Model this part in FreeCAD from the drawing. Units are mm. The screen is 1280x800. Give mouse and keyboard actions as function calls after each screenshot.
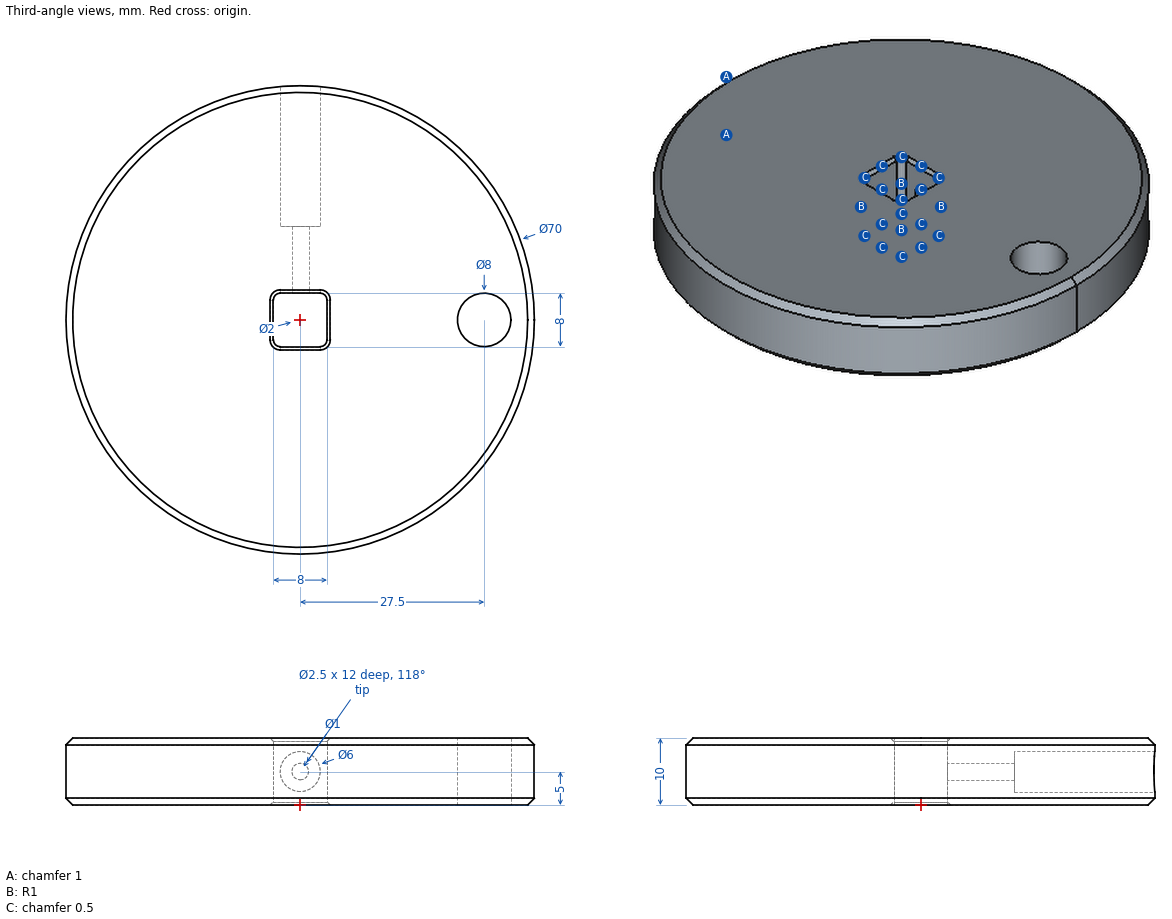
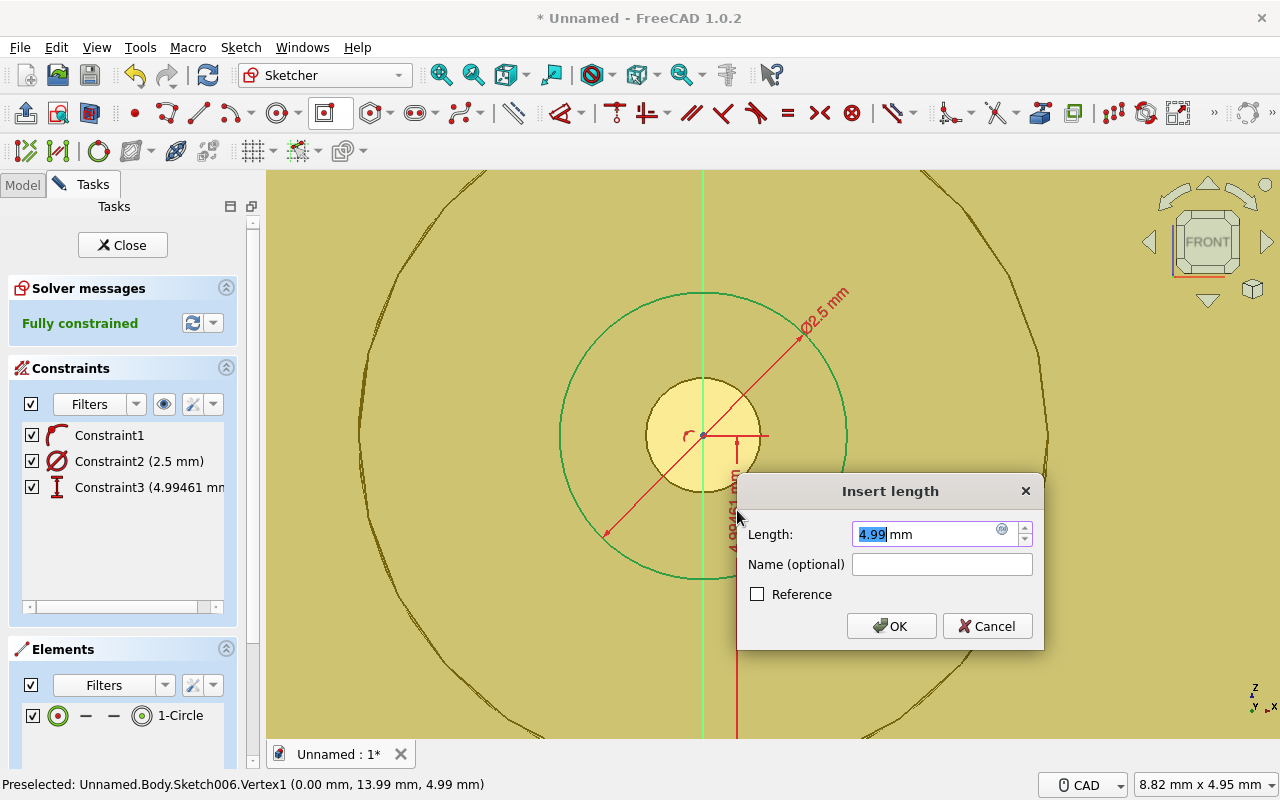
text(5)
key(Return)
key(Escape)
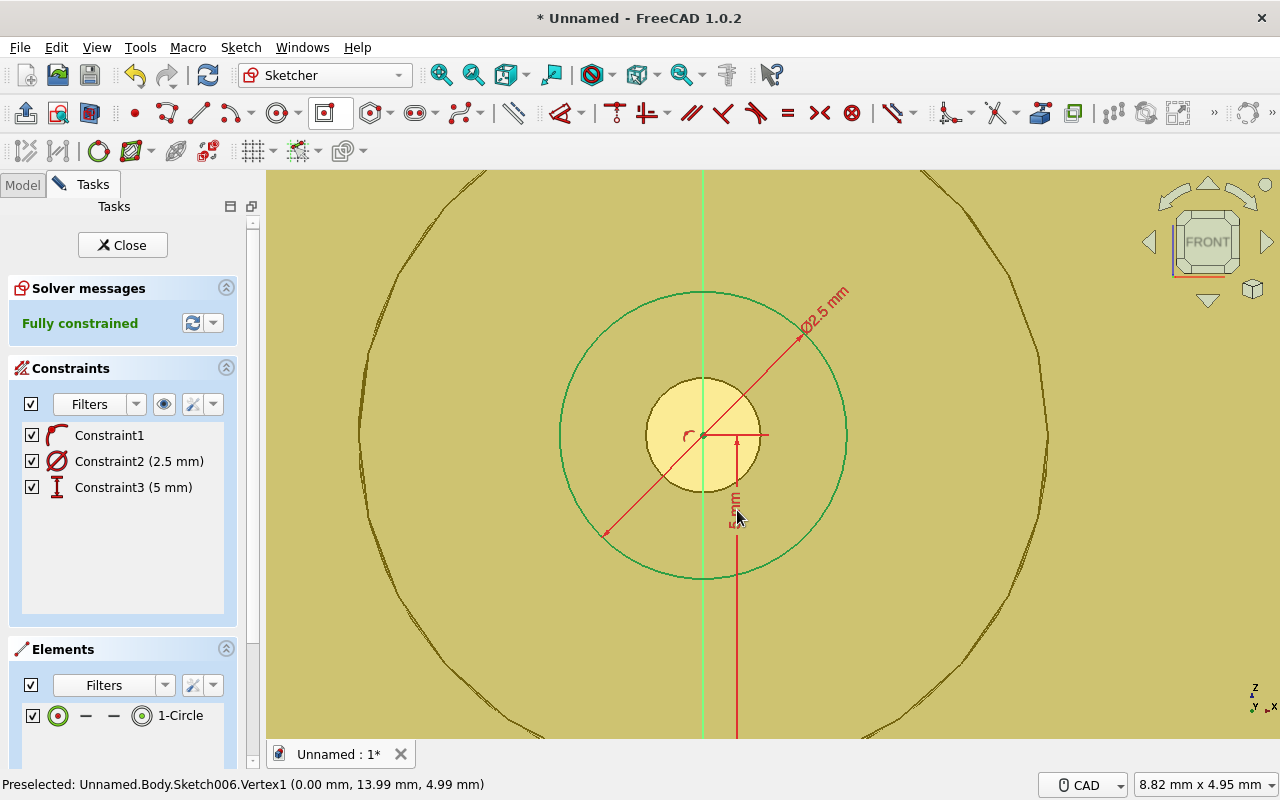
click(123, 245)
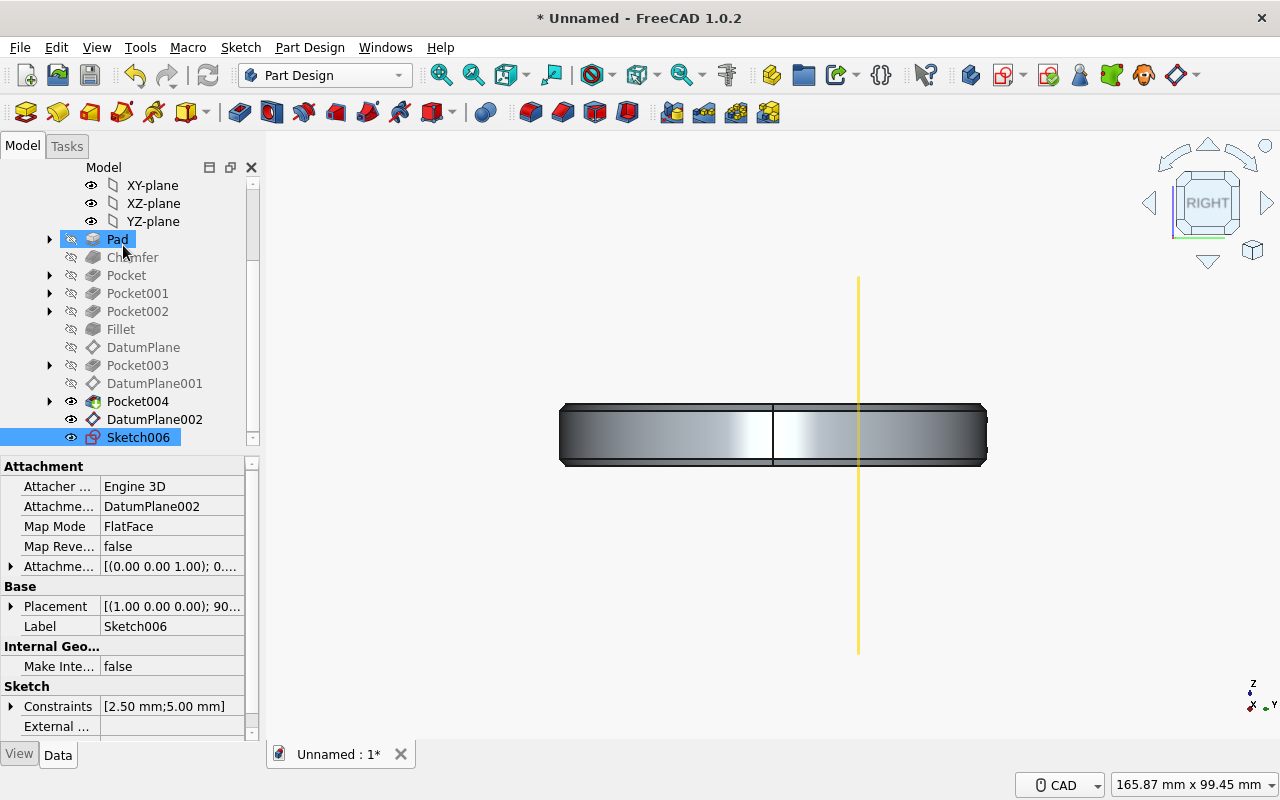
click(272, 112)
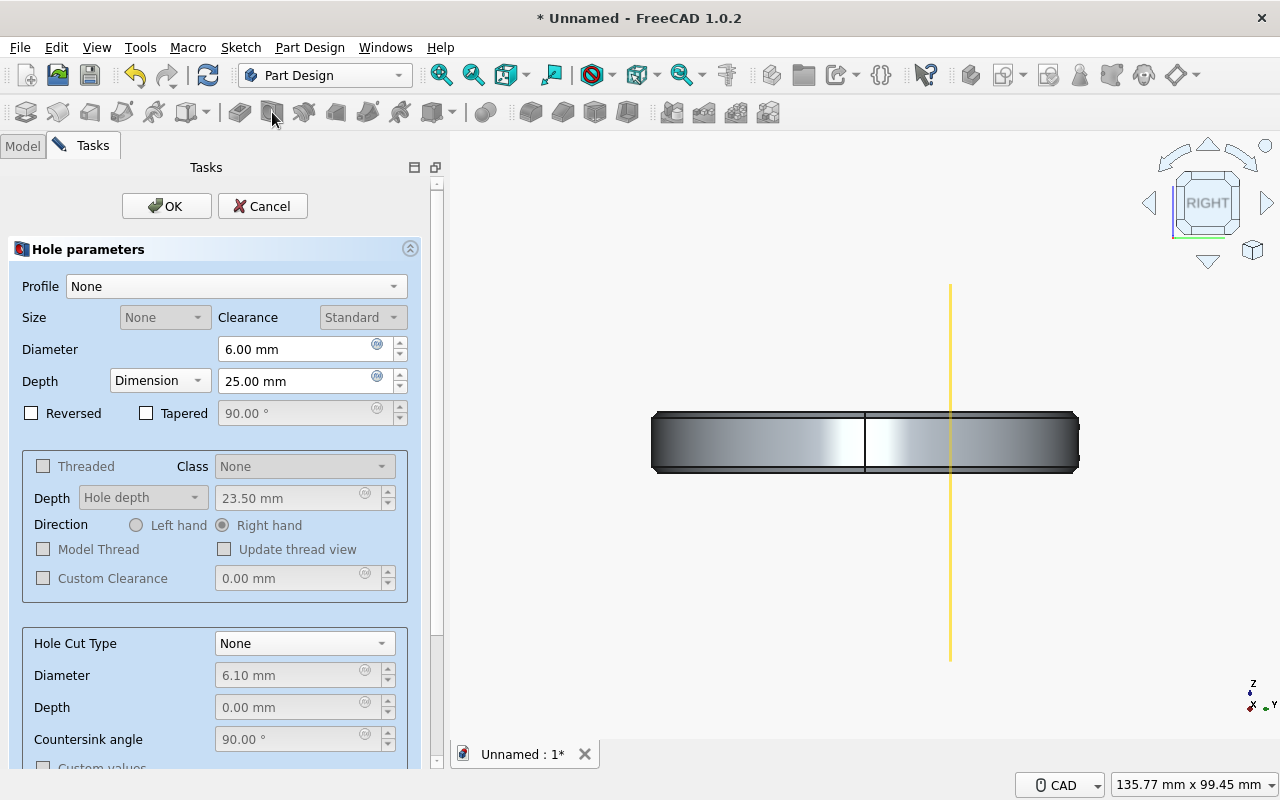
triple_click(305, 349)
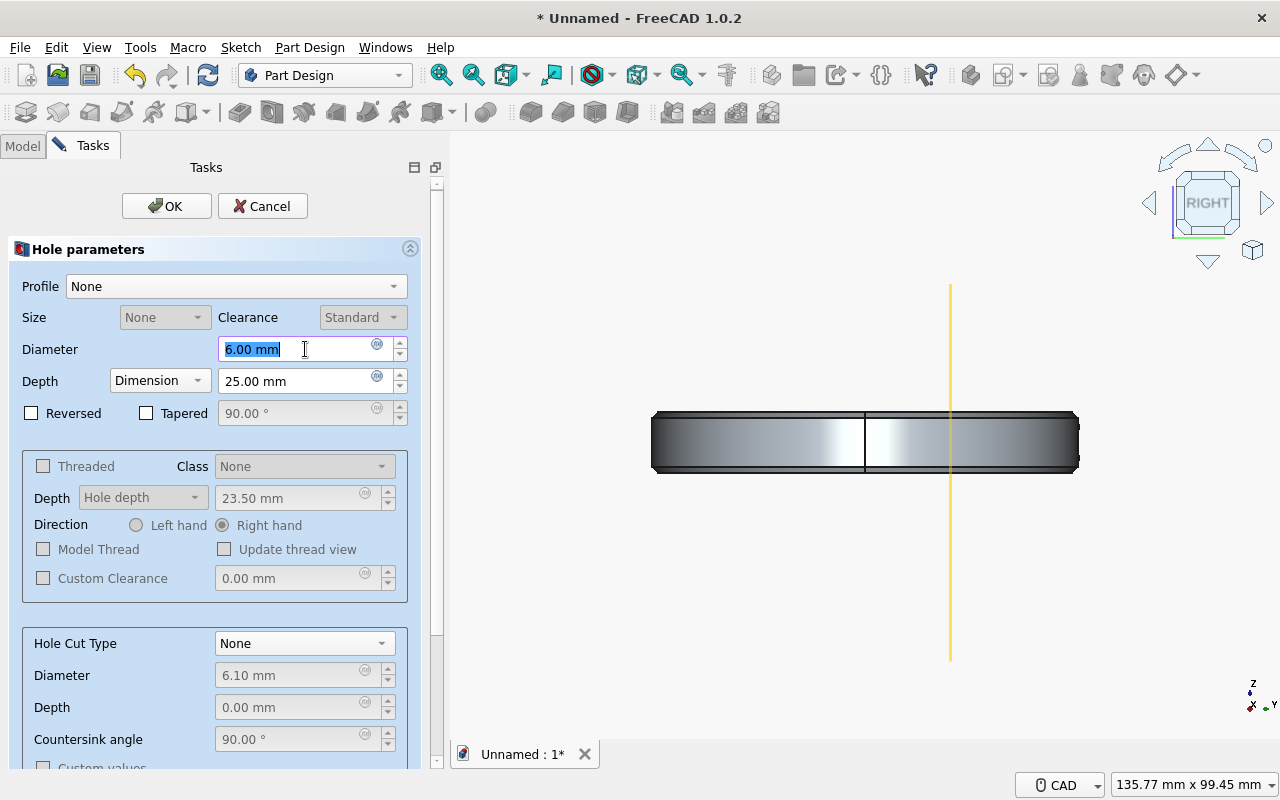
text(2.5)
key(Tab)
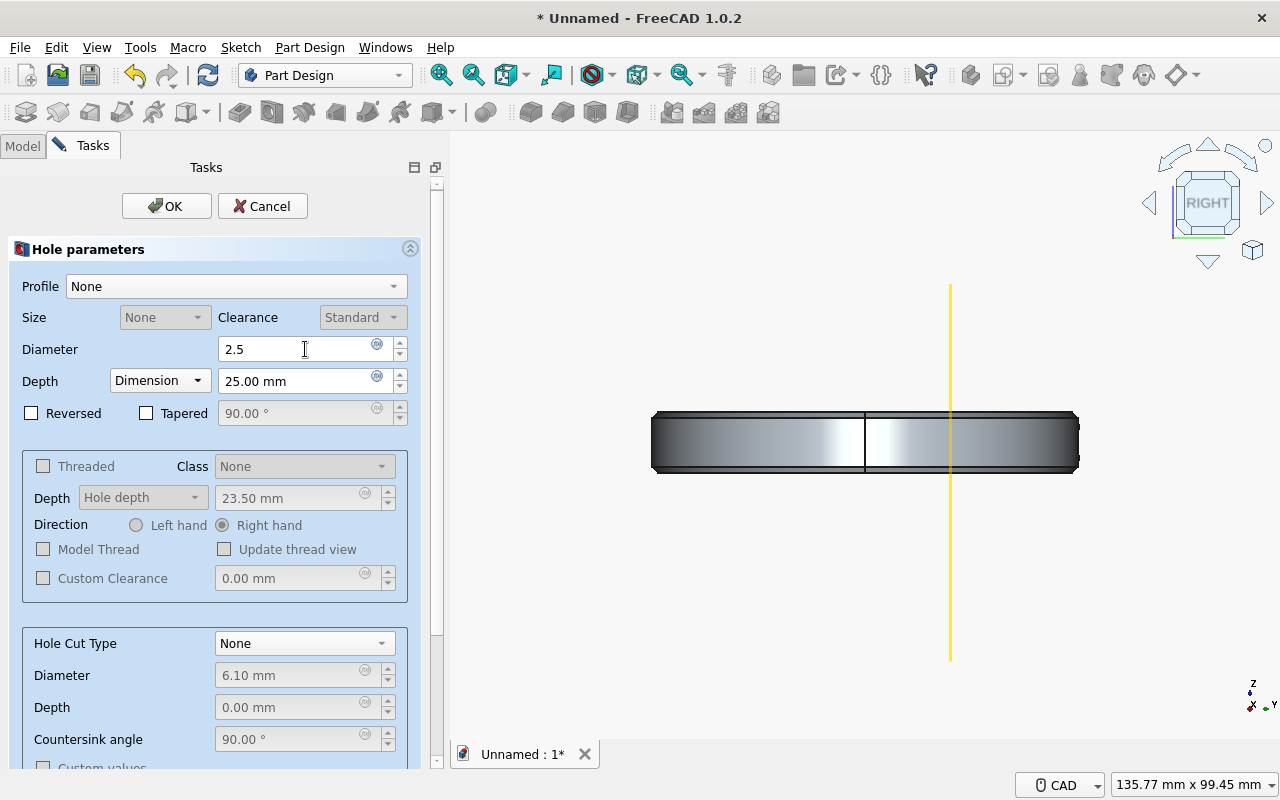
triple_click(305, 381)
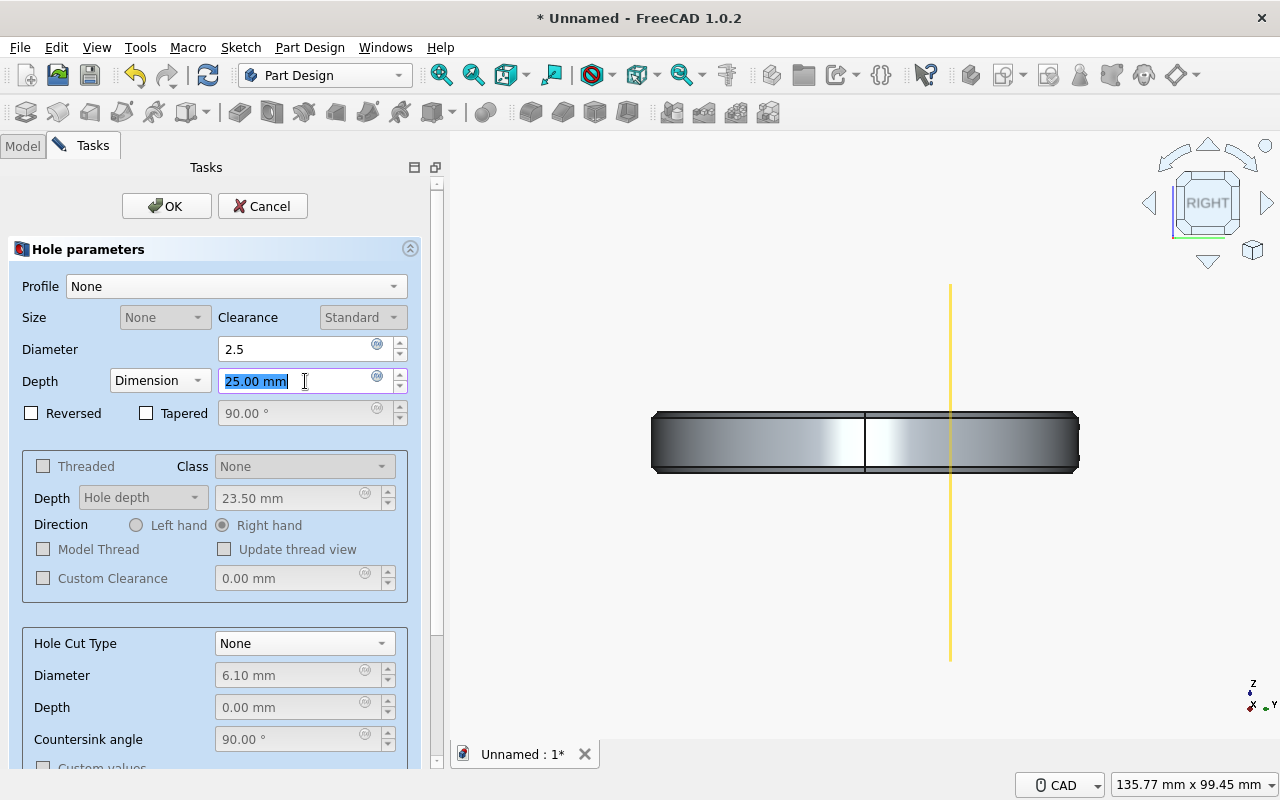
text(12)
key(Tab)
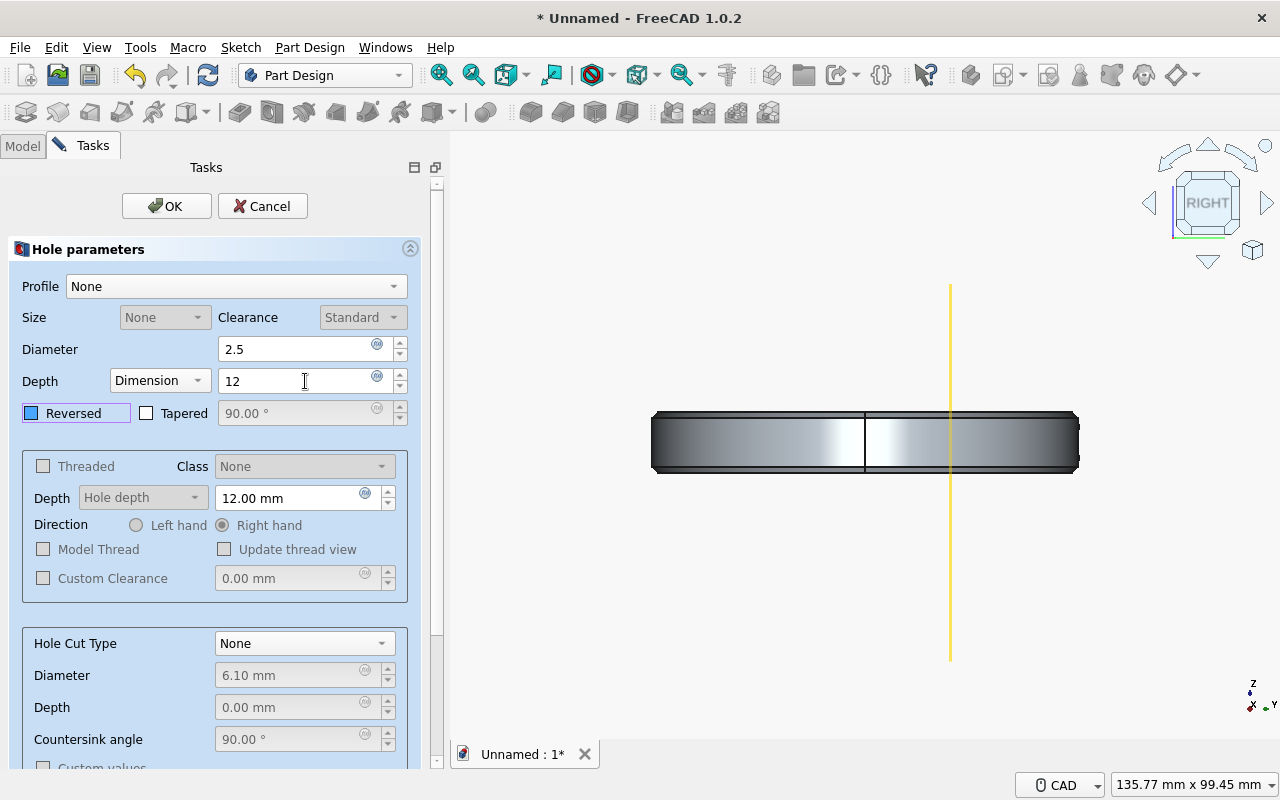
click(30, 413)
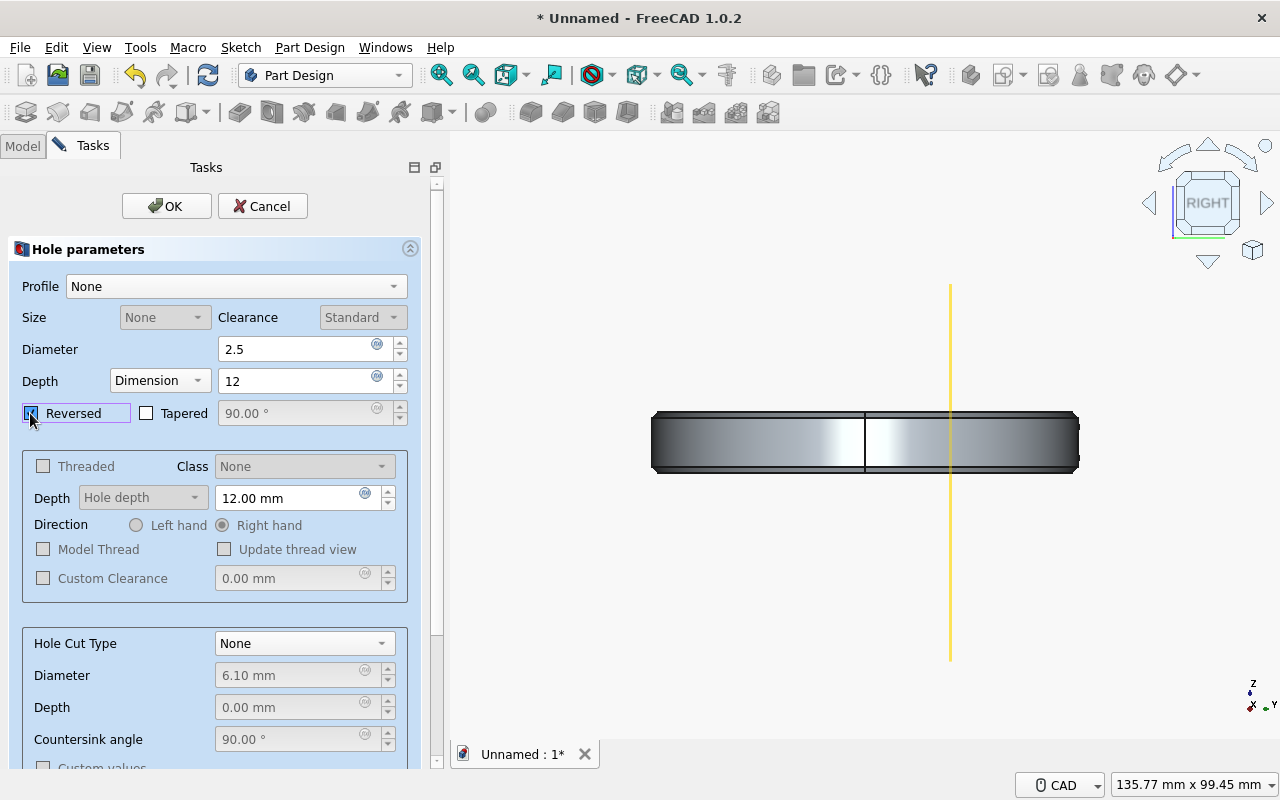
click(167, 206)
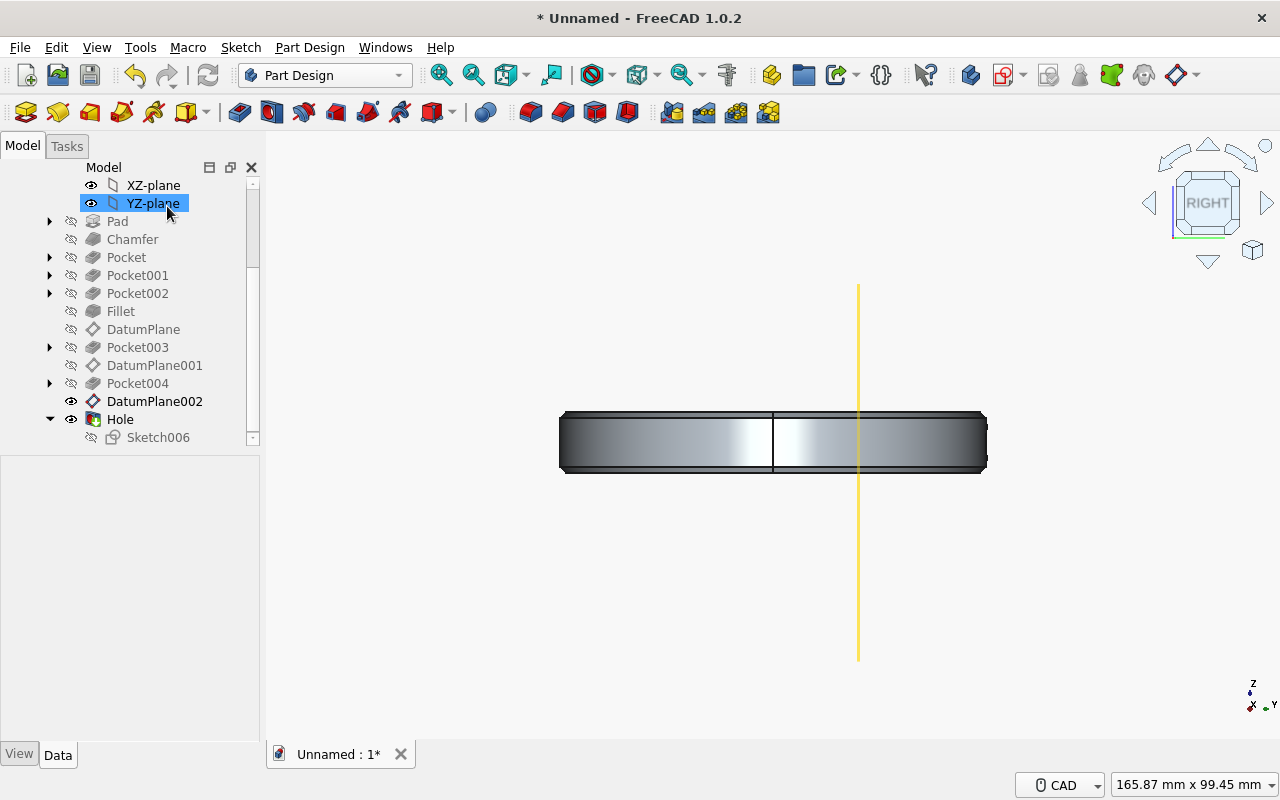
click(116, 401)
key(space)